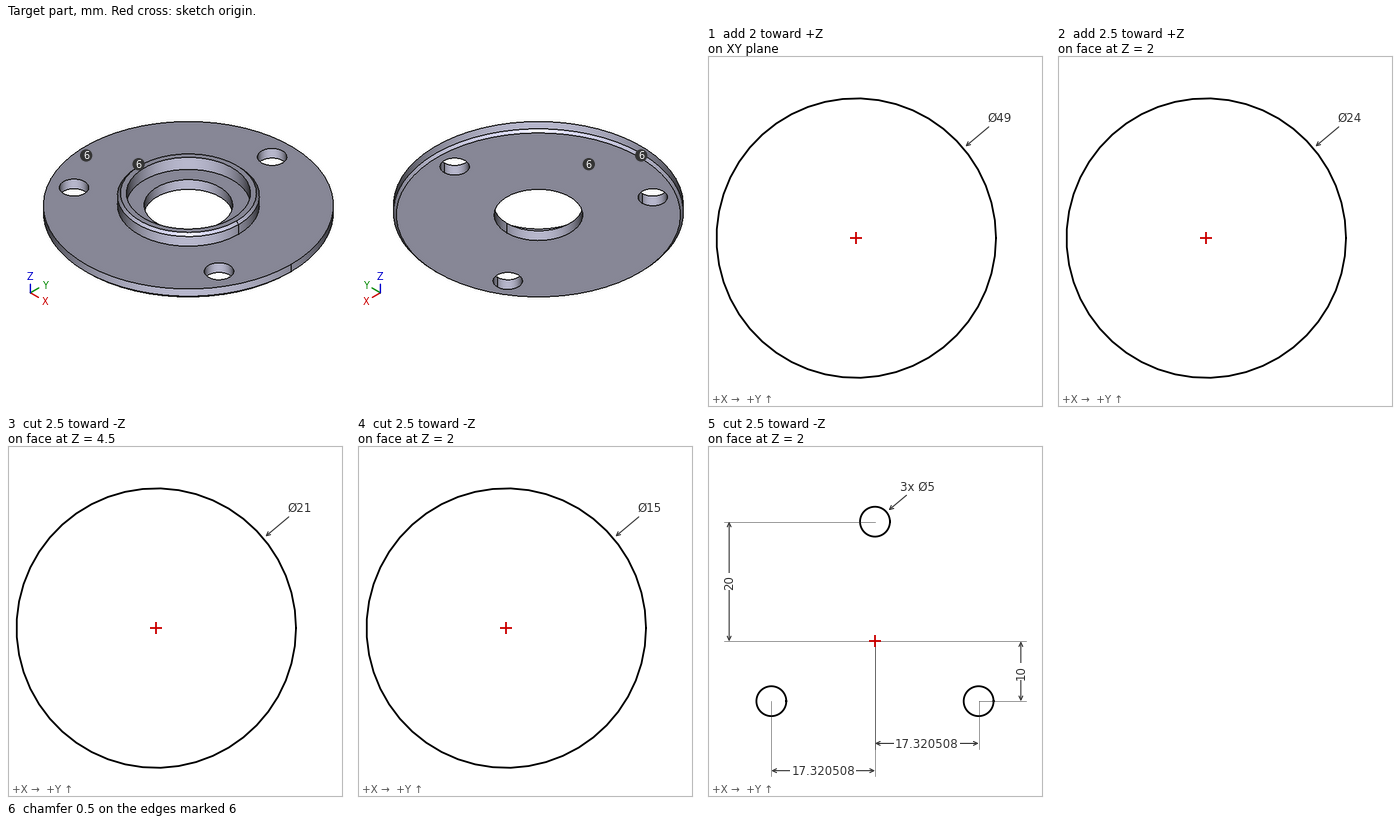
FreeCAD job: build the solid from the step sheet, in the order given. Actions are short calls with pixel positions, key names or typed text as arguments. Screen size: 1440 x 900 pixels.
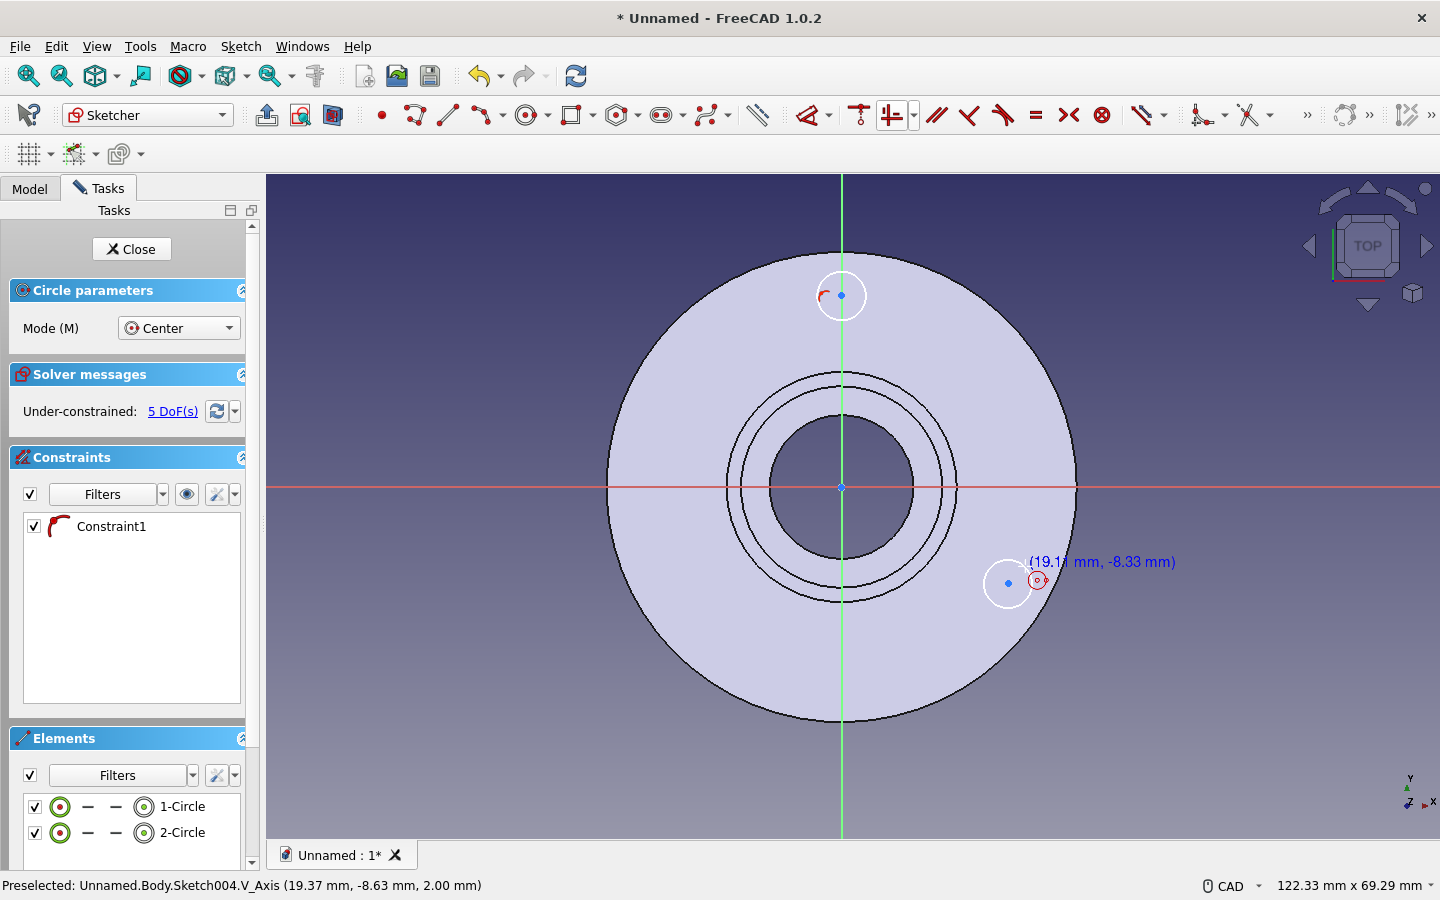
click(675, 583)
click(692, 566)
key(Escape)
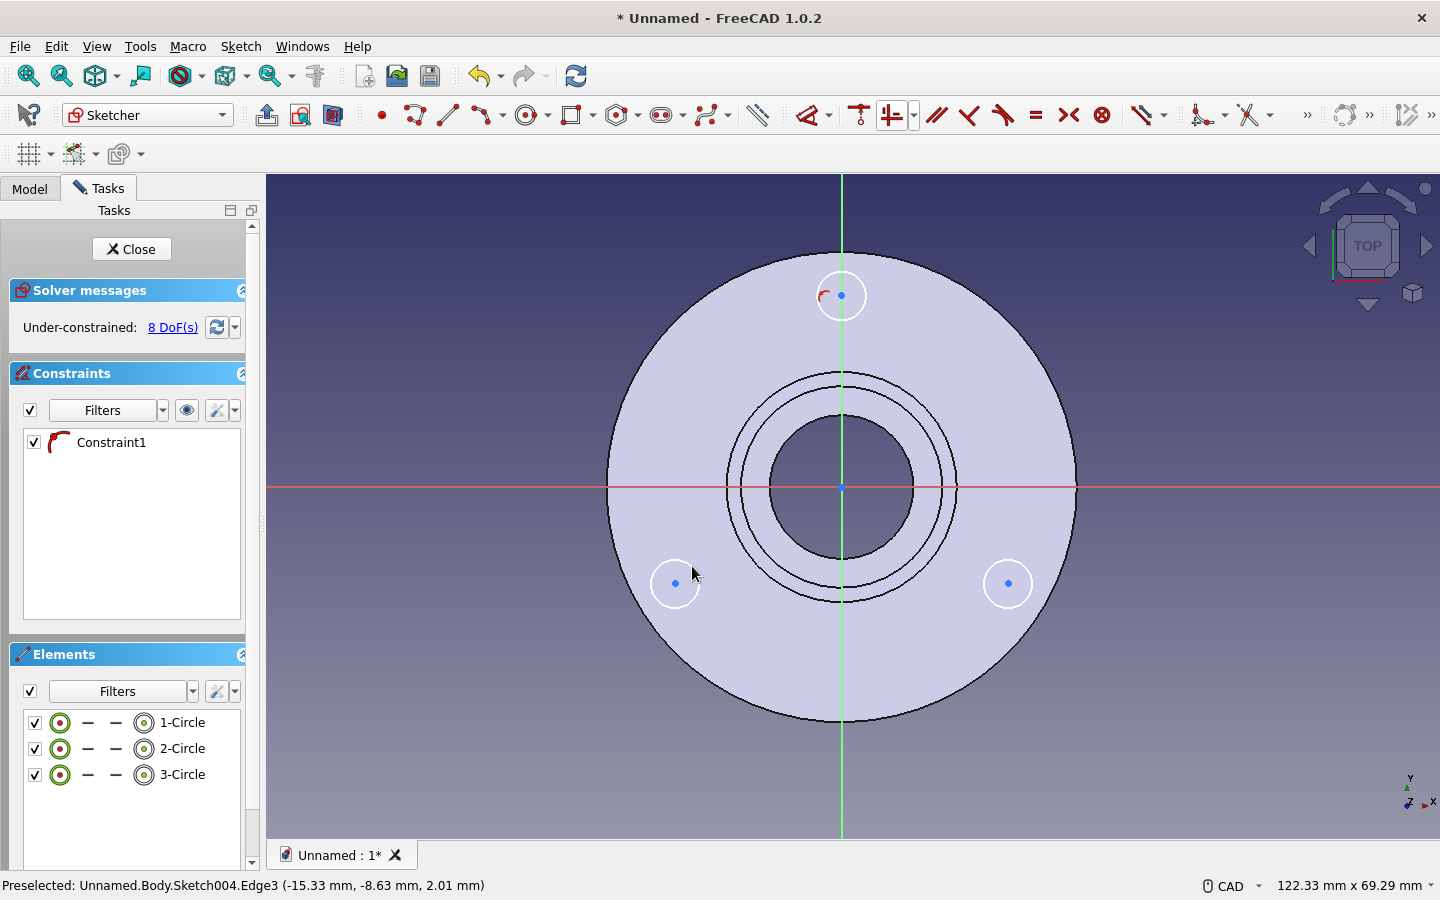
click(859, 279)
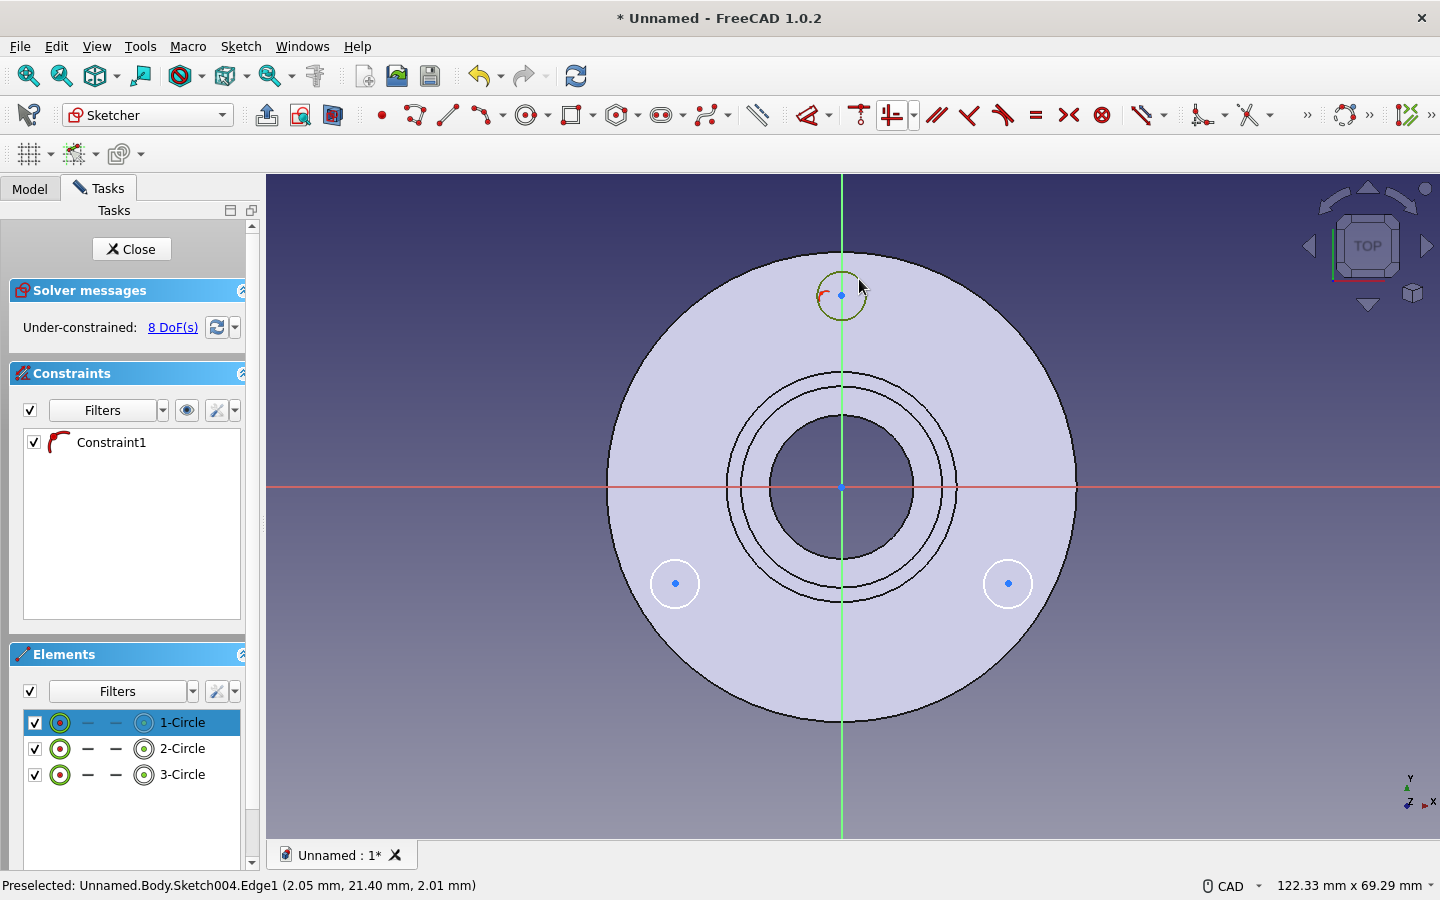
click(1025, 567)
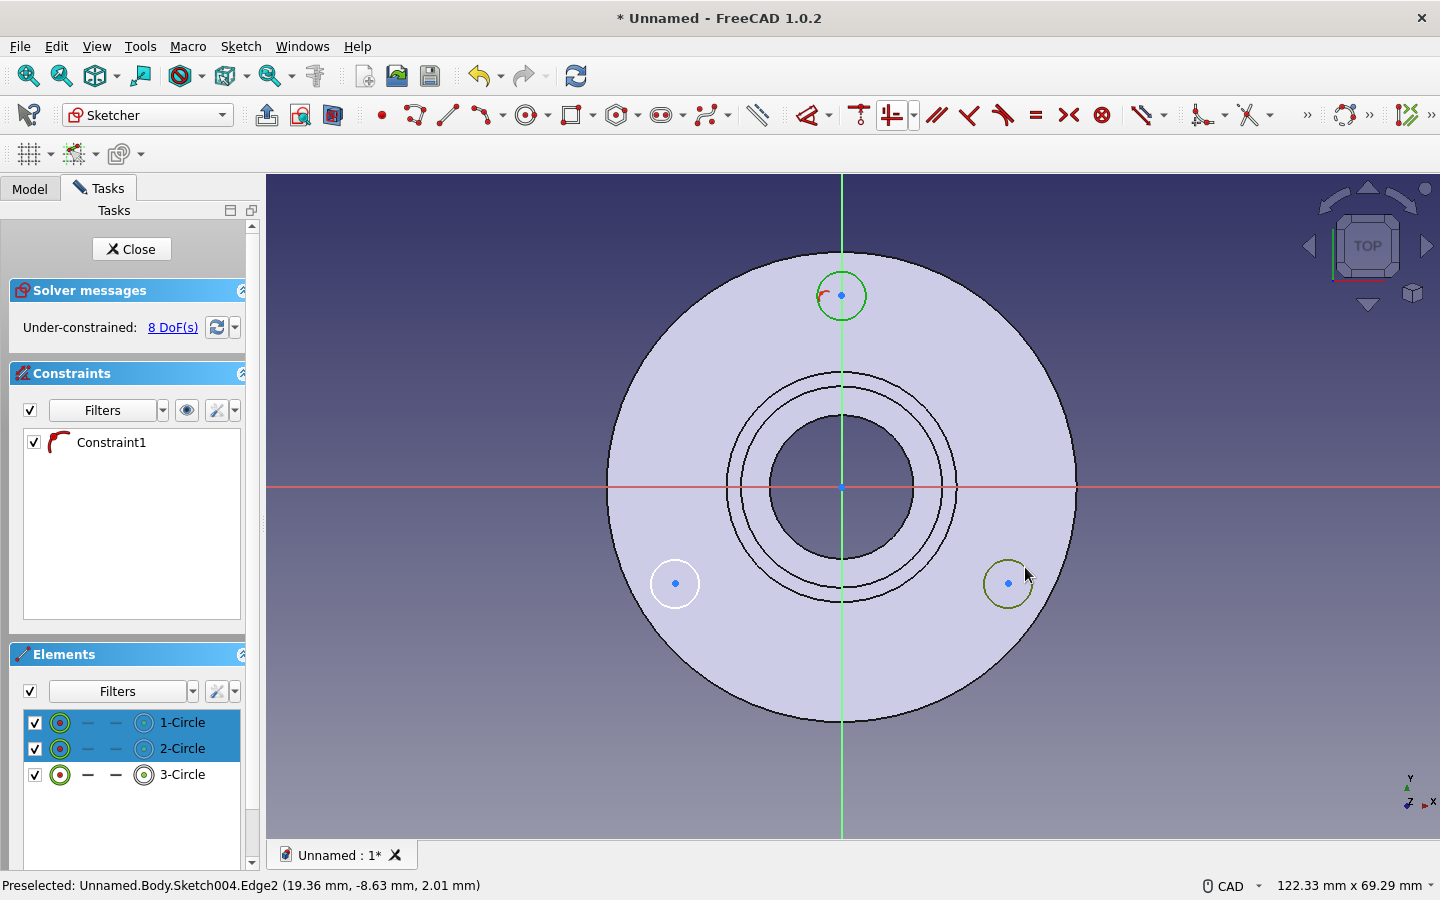
click(692, 567)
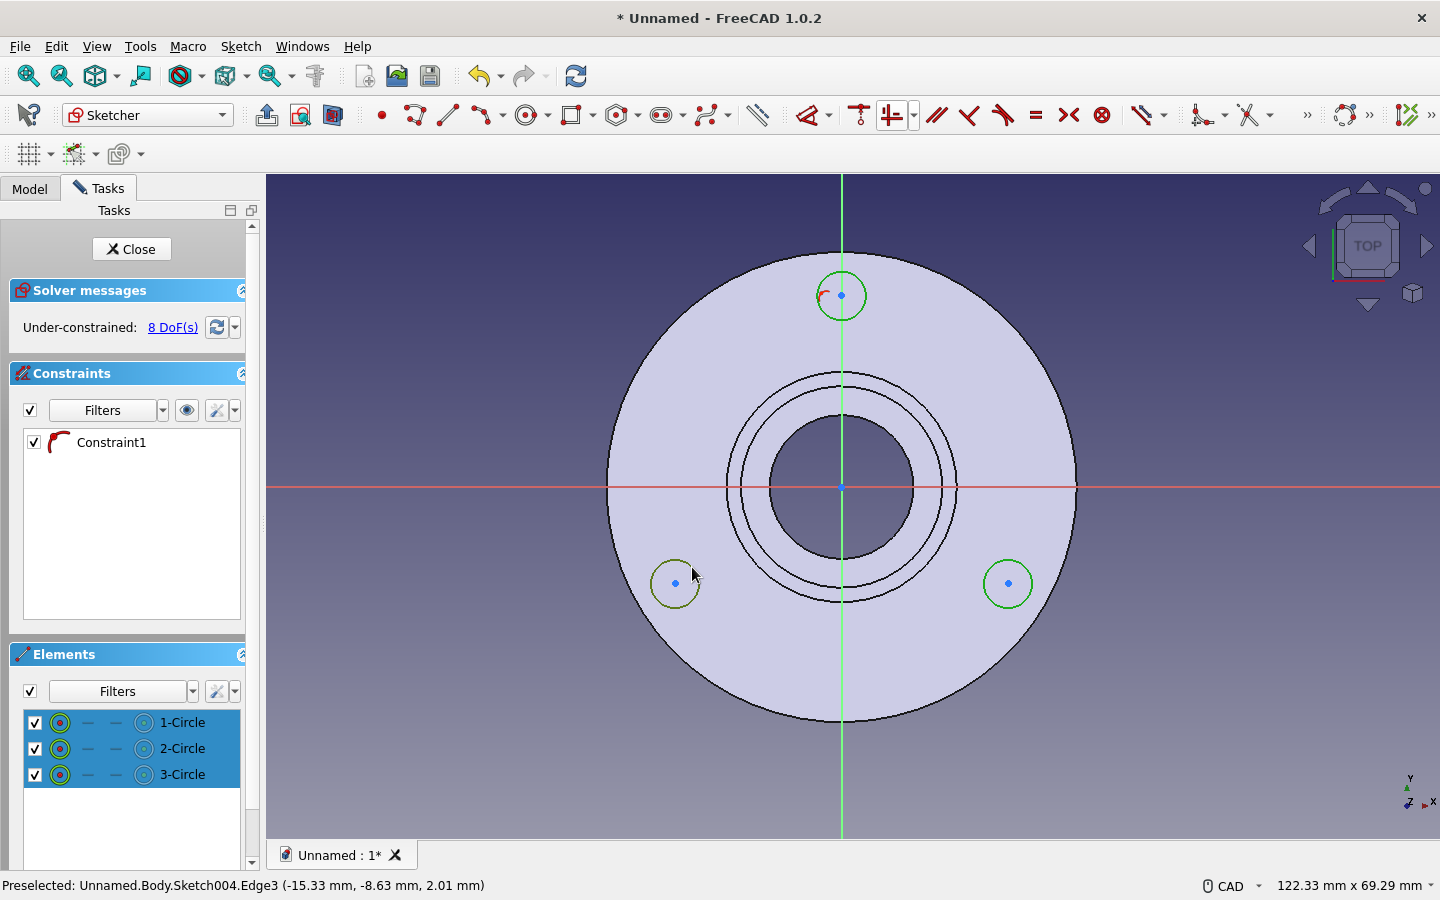
click(1036, 116)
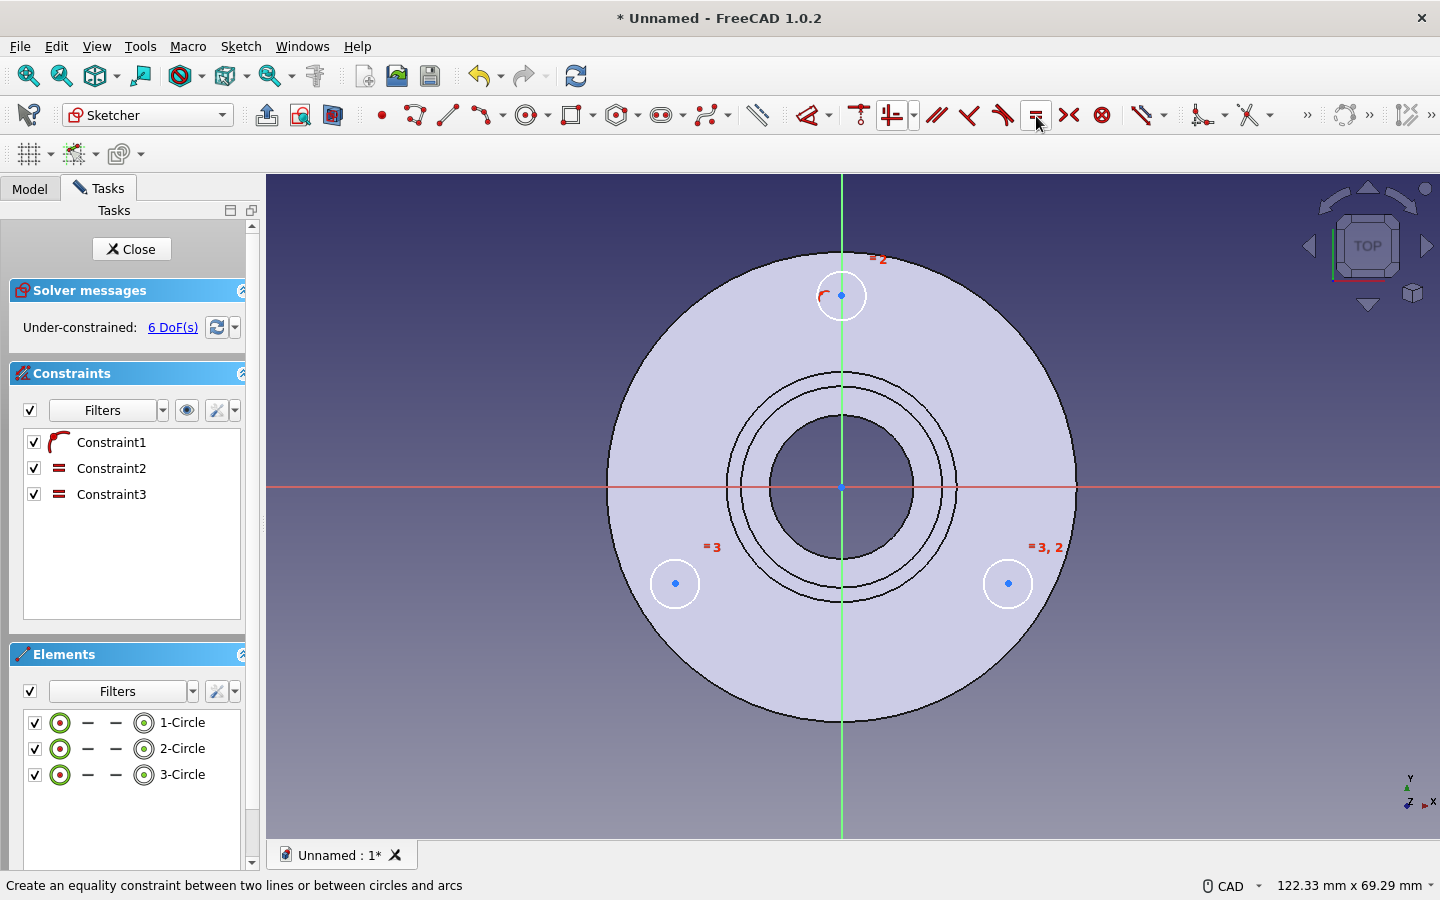
click(1008, 584)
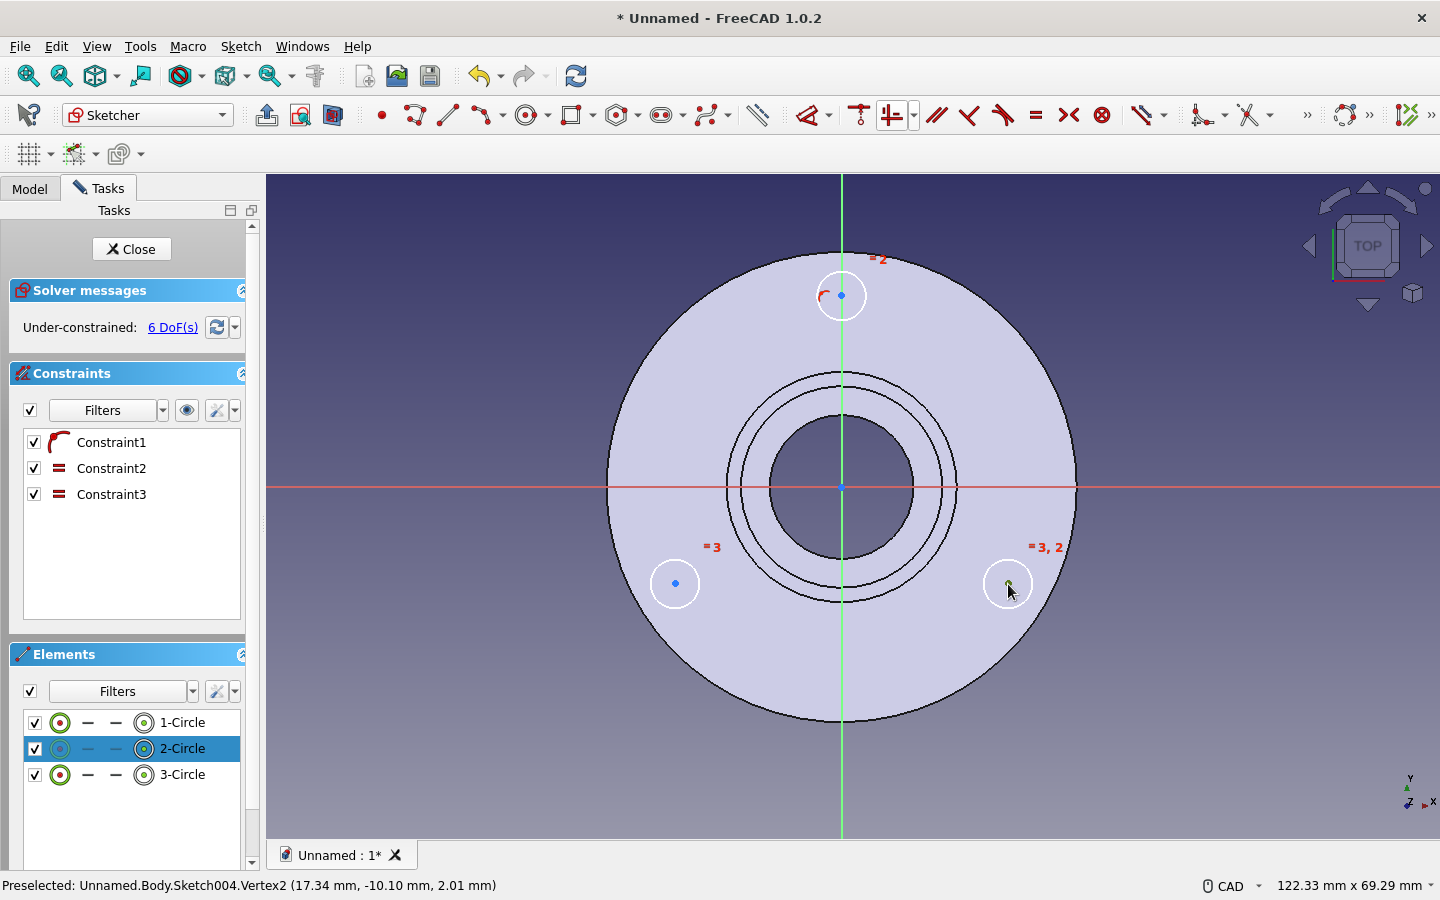
click(675, 584)